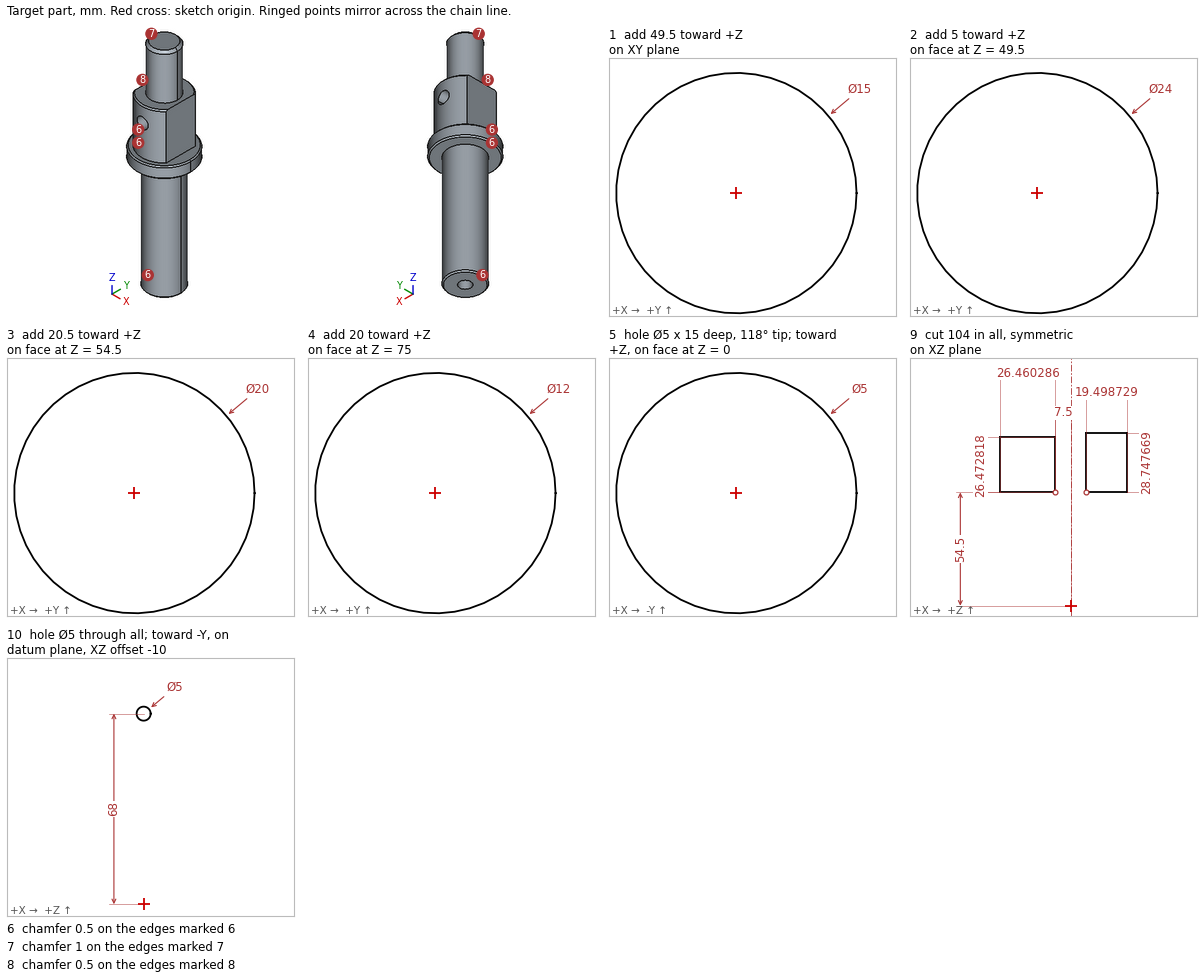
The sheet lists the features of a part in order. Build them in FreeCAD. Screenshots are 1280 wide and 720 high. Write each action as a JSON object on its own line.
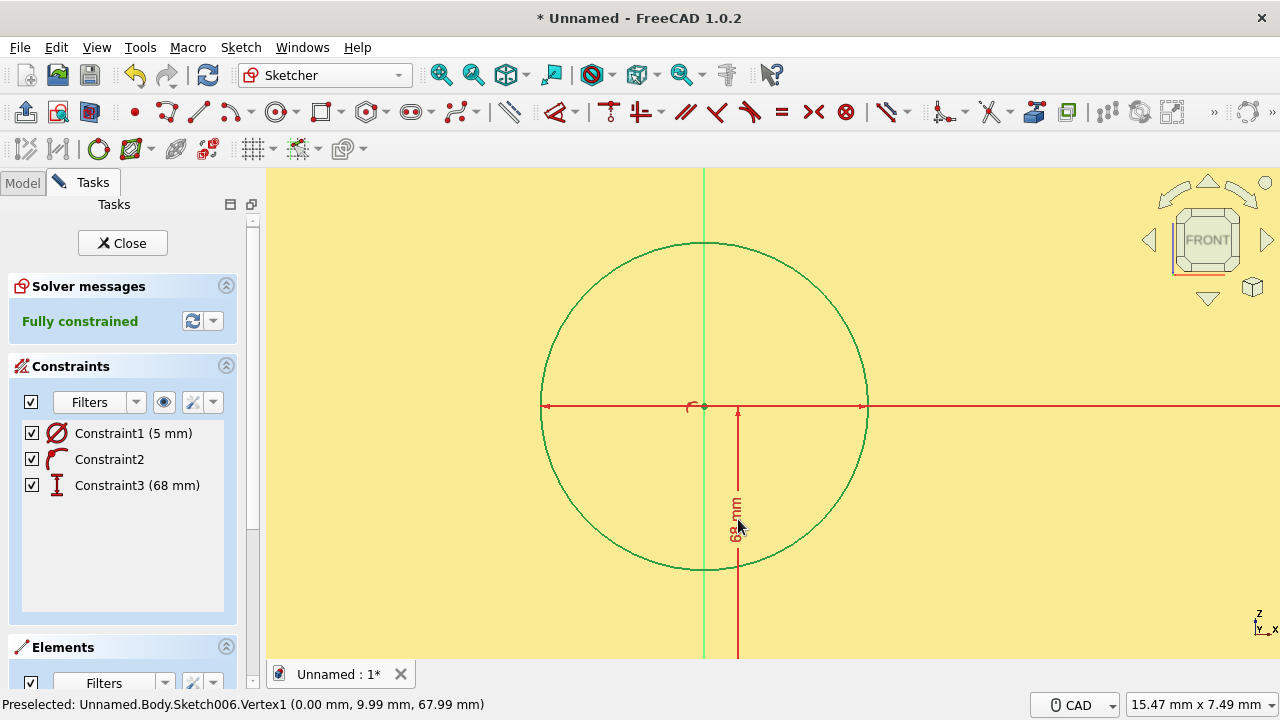
{"action": "left_click", "coordinate": [123, 243]}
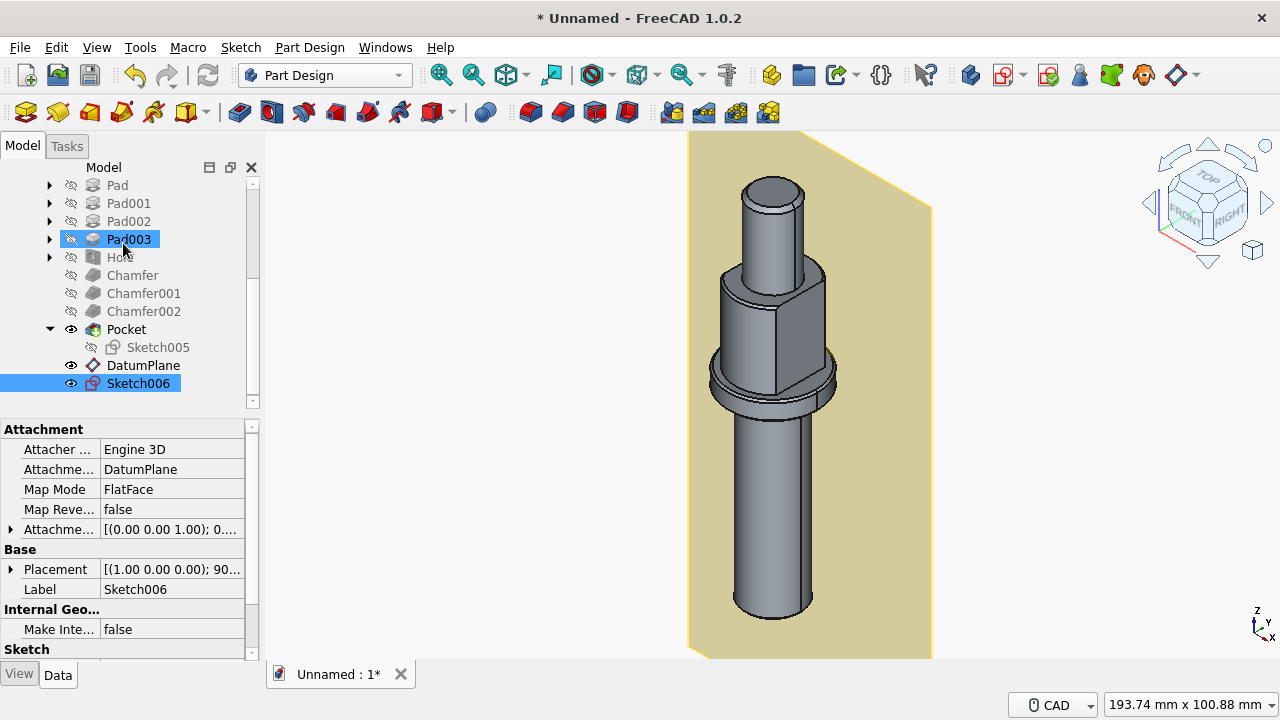
{"action": "left_click", "coordinate": [272, 112]}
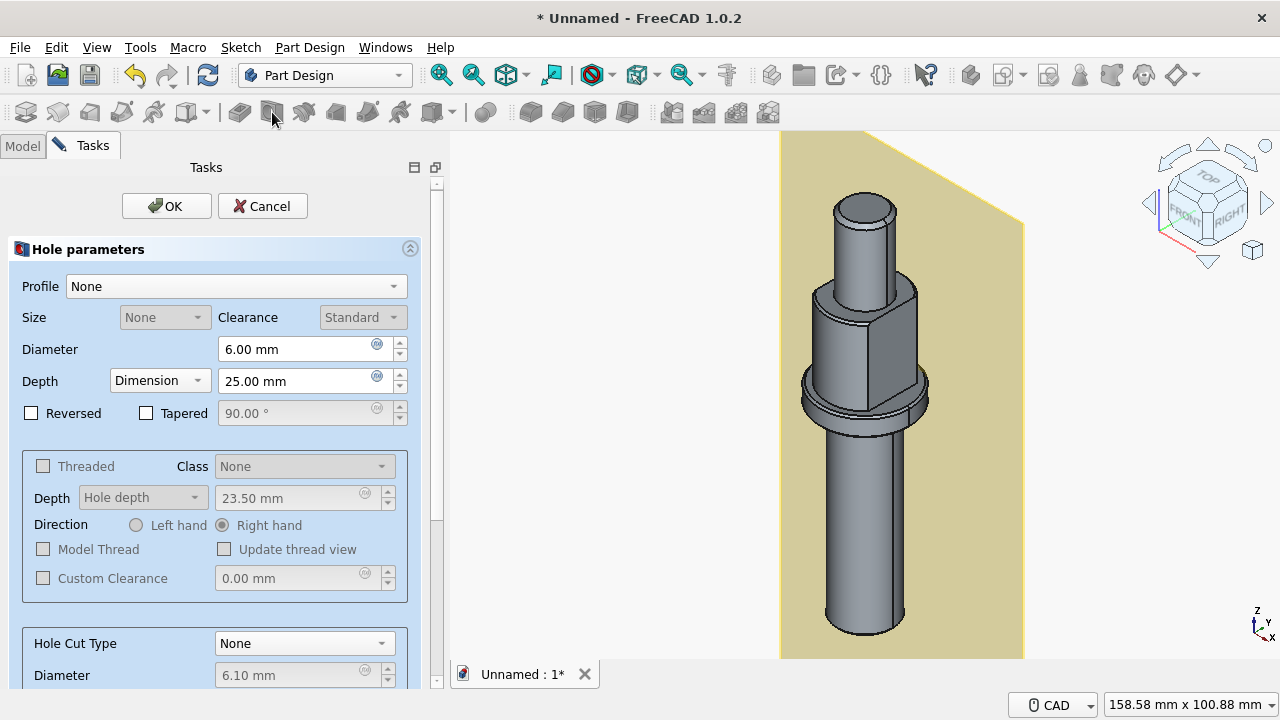
{"action": "triple_click", "coordinate": [305, 349]}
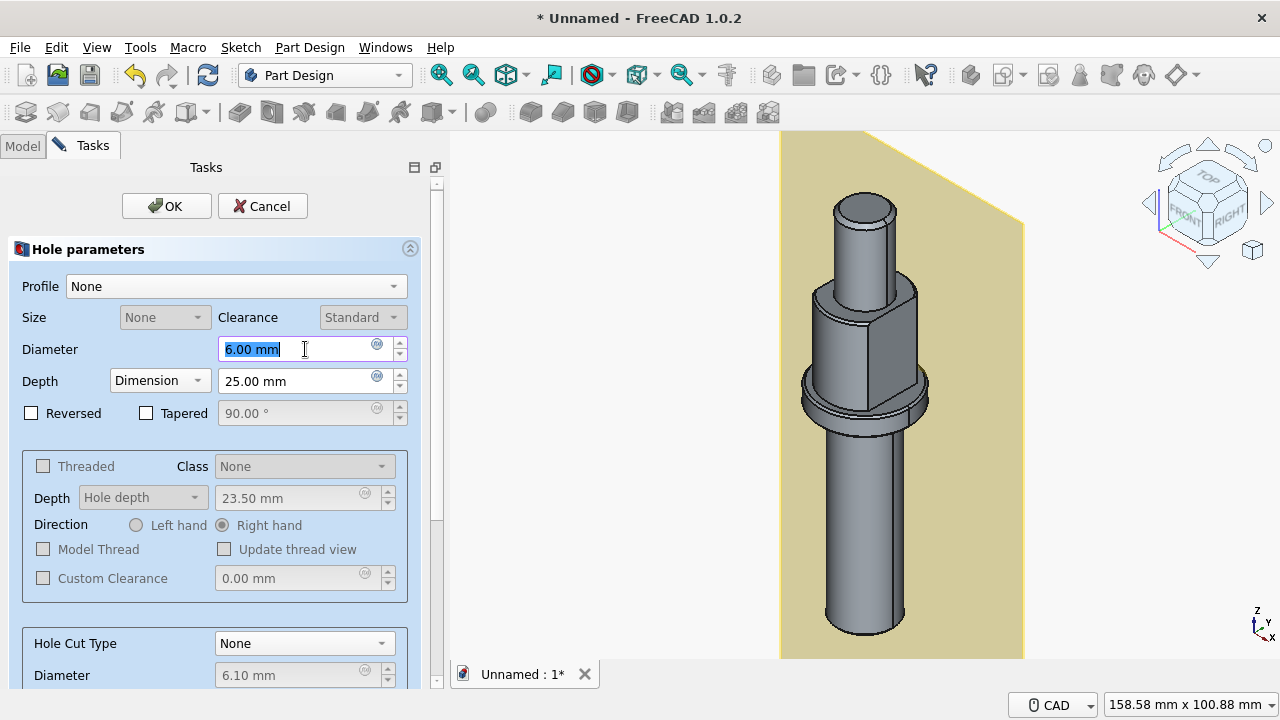
{"action": "type", "text": "5"}
{"action": "key", "text": "Tab"}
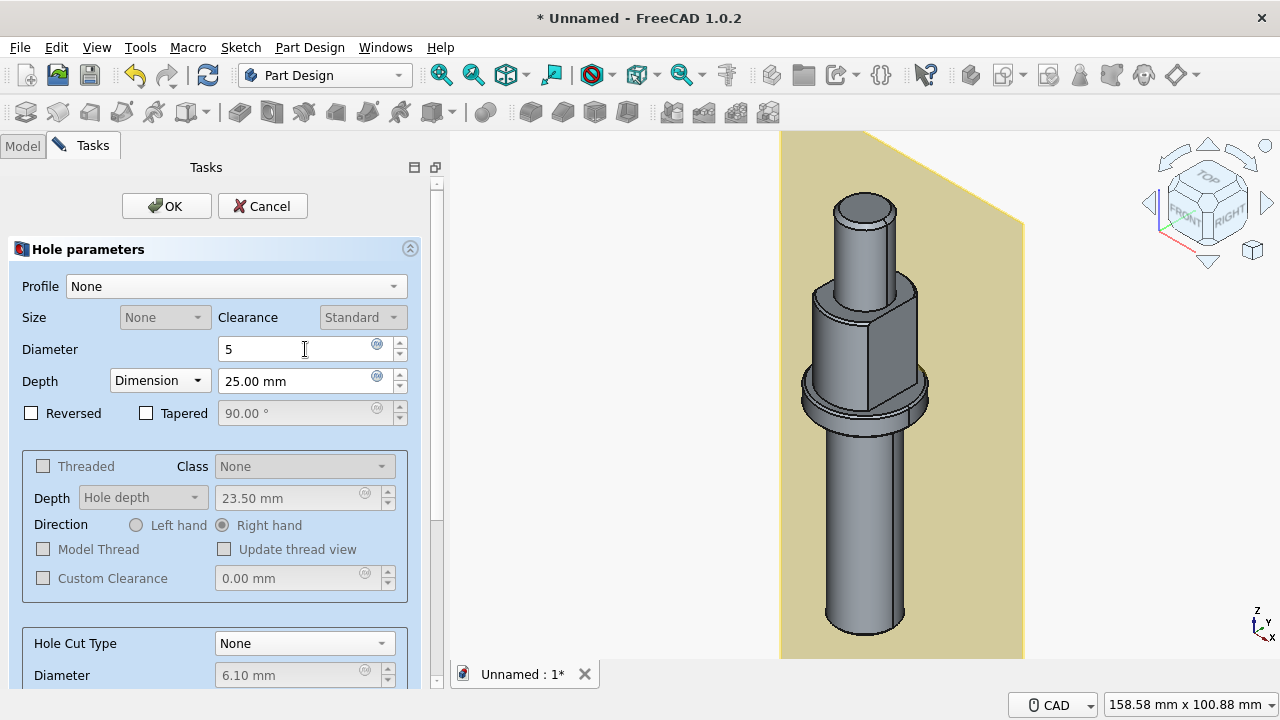
{"action": "left_click", "coordinate": [161, 380]}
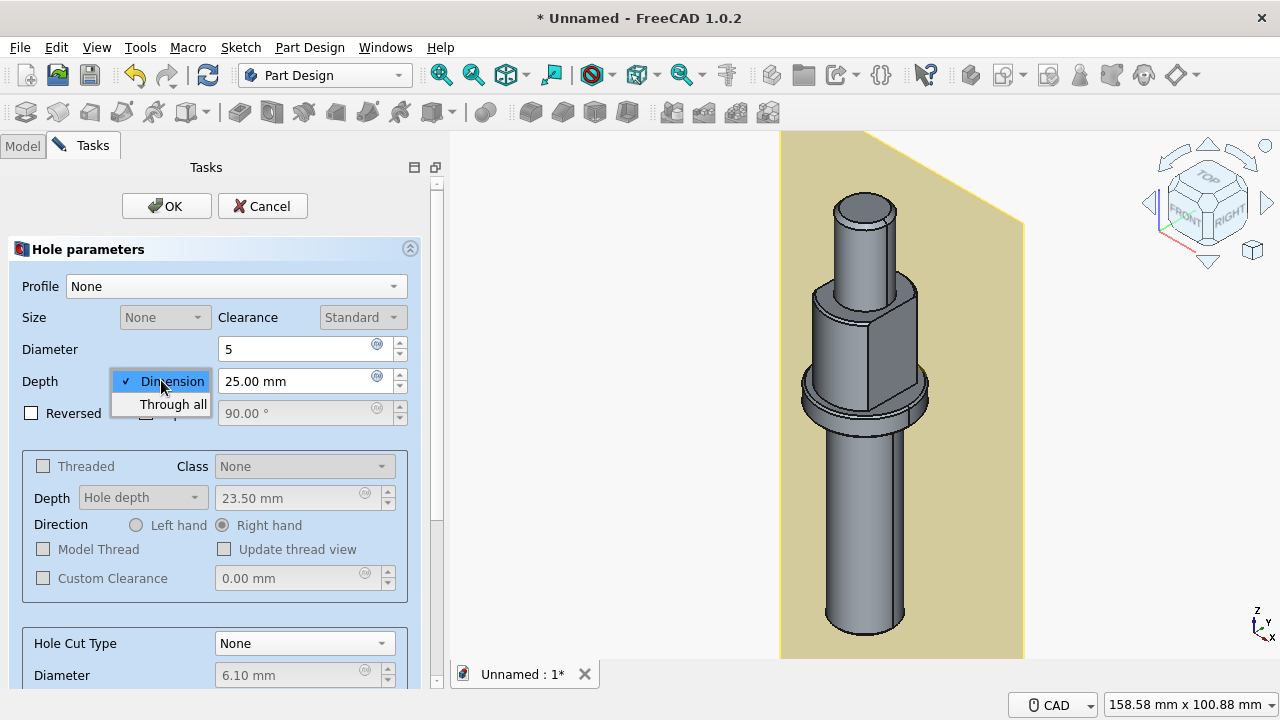
{"action": "left_click", "coordinate": [160, 404]}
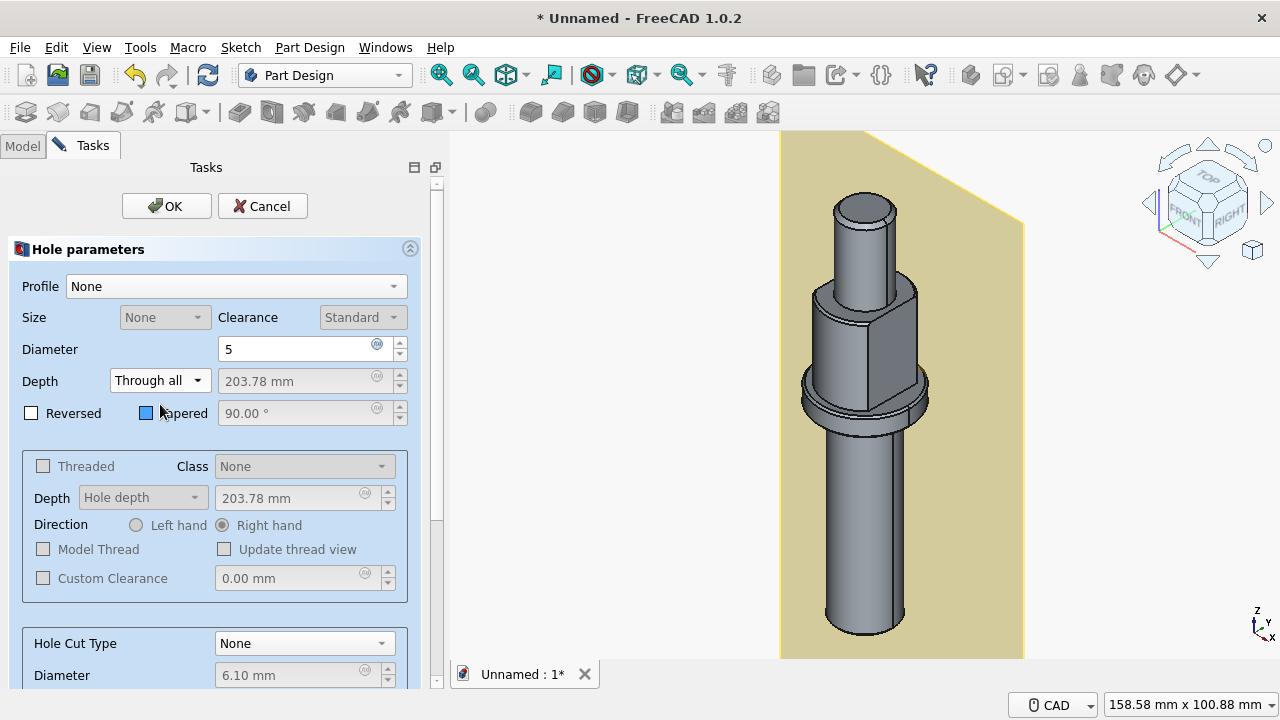
{"action": "left_click", "coordinate": [30, 413]}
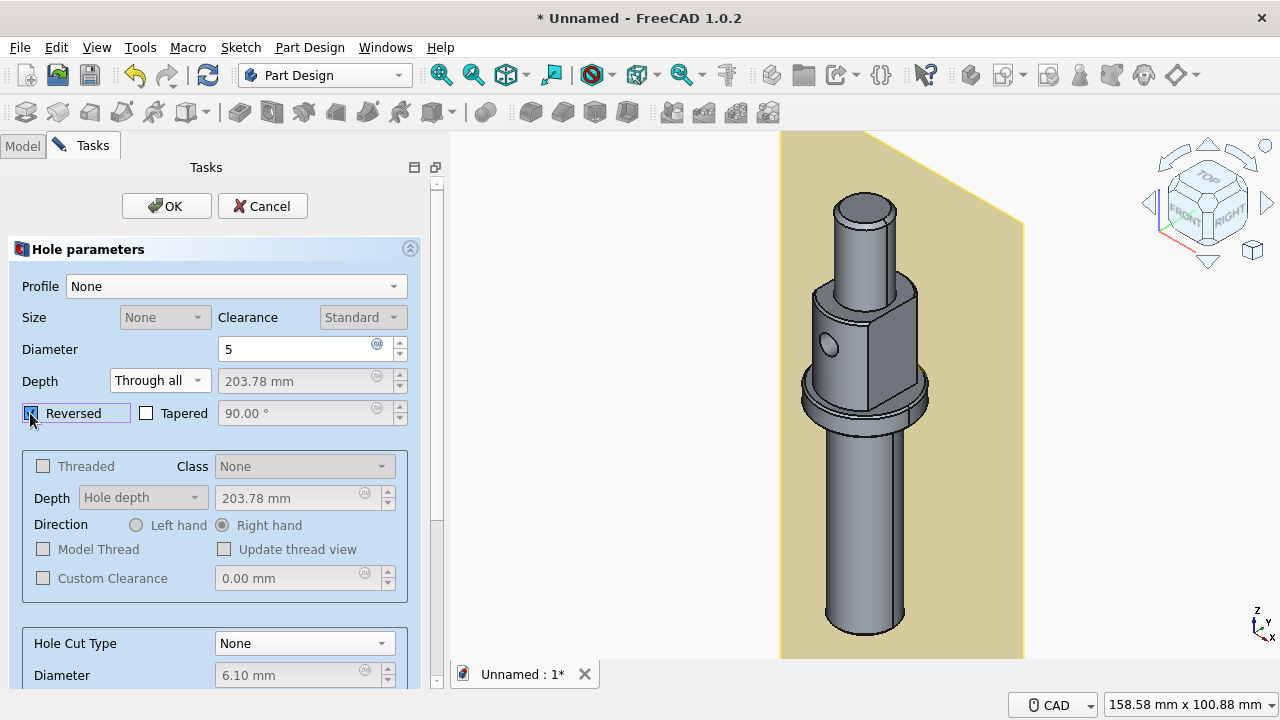
{"action": "left_click", "coordinate": [167, 206]}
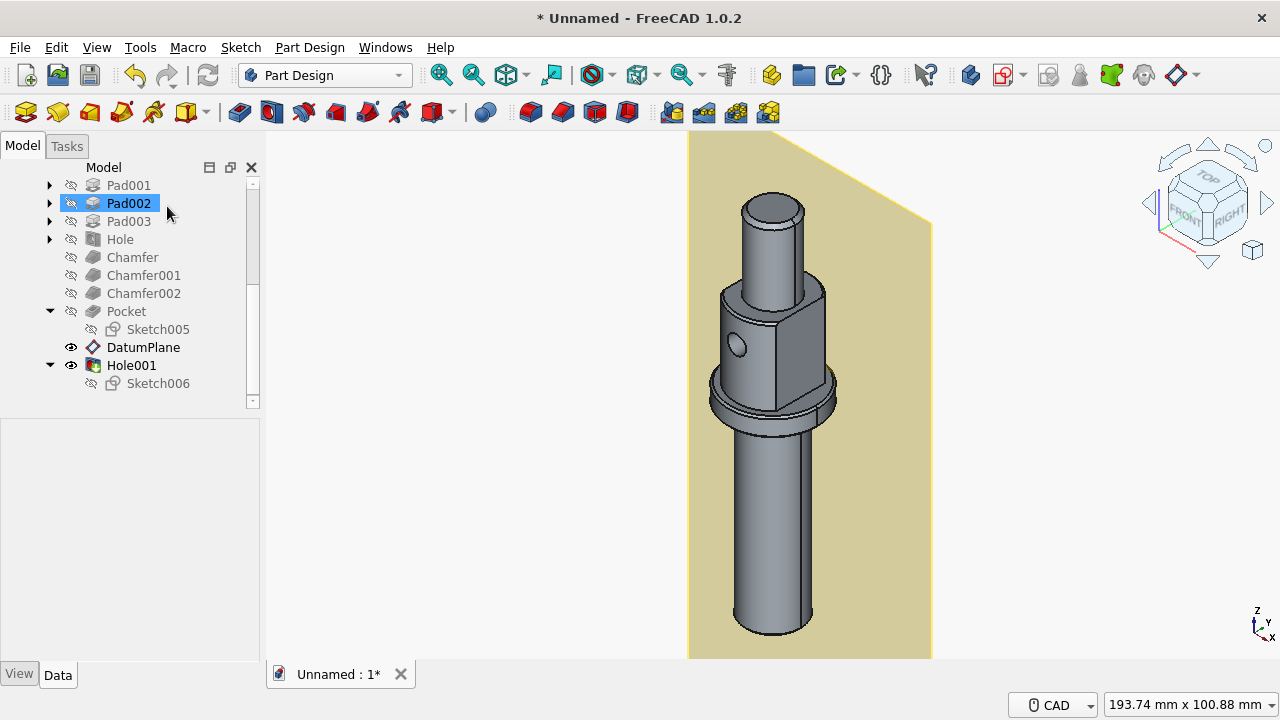
{"action": "left_click", "coordinate": [116, 347]}
{"action": "key", "text": "space"}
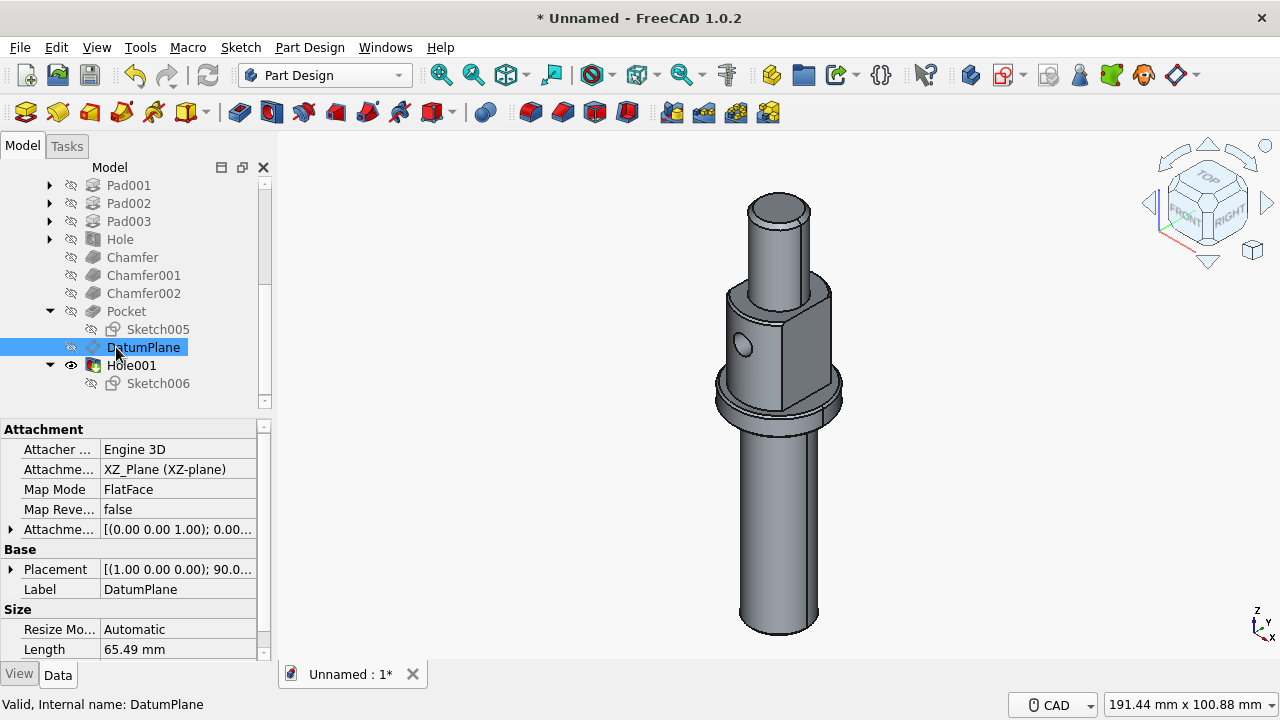
{"action": "key", "text": "v f"}